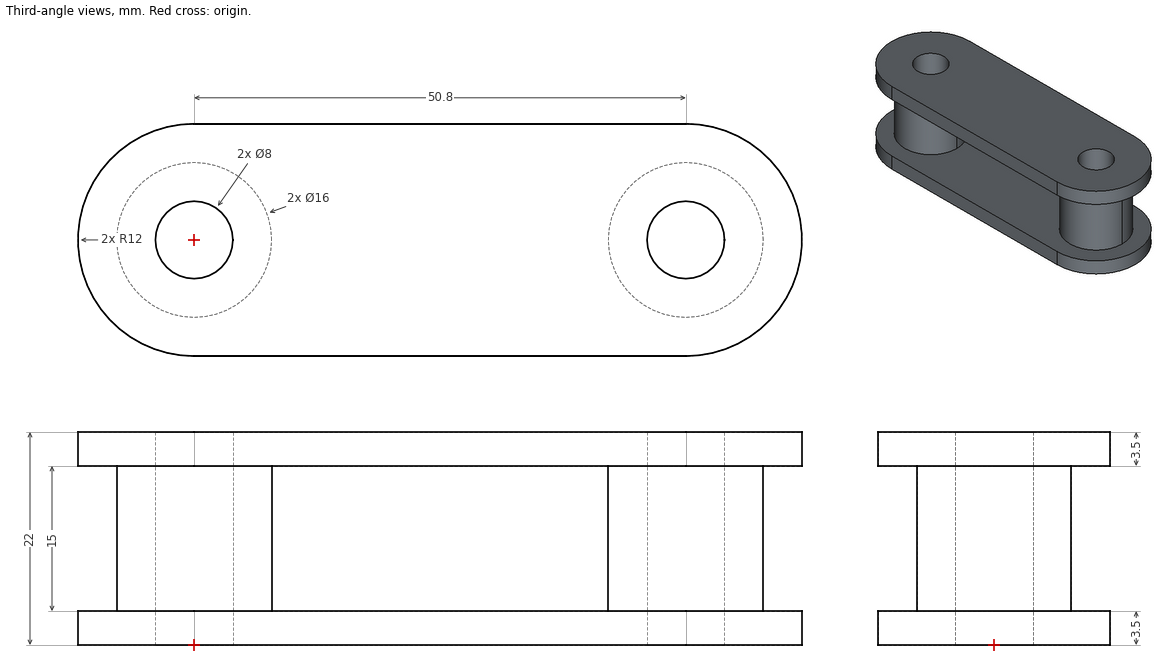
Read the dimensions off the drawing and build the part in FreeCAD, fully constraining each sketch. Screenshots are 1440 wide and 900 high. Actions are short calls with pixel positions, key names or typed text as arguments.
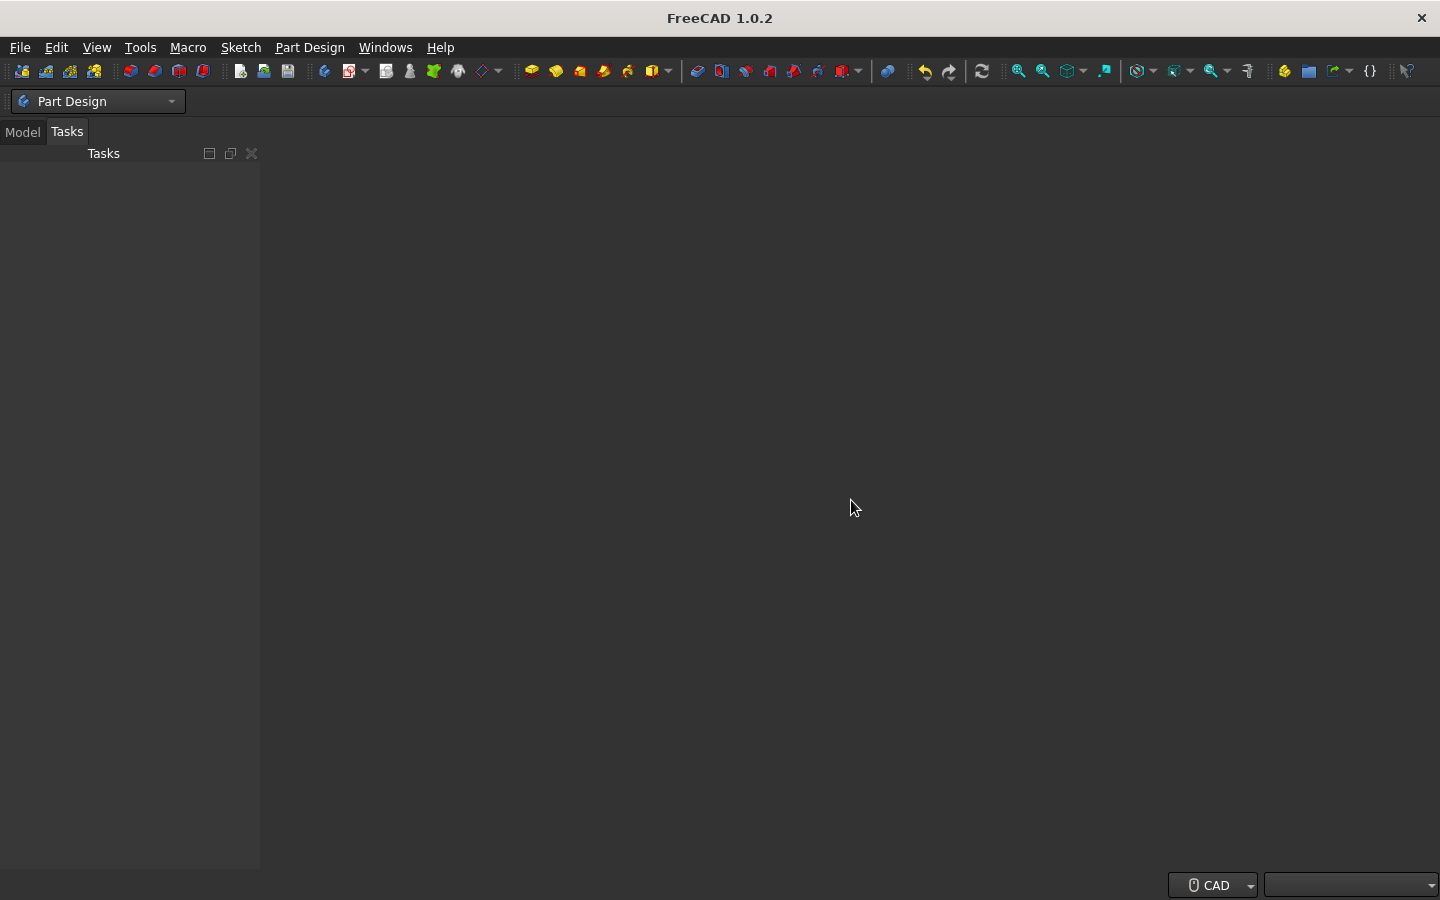
key(ctrl+n)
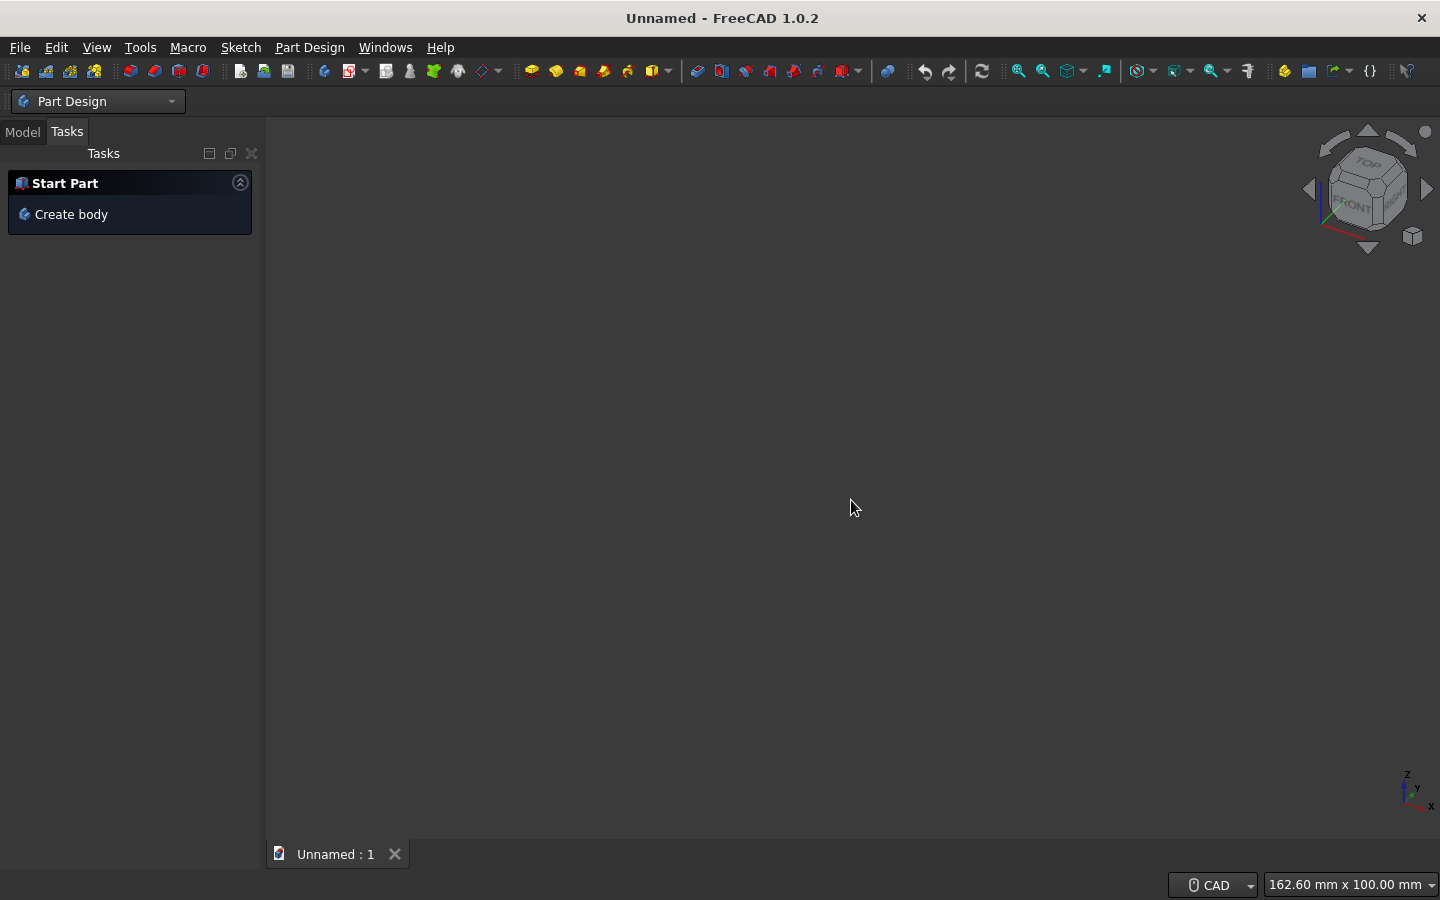
click(350, 72)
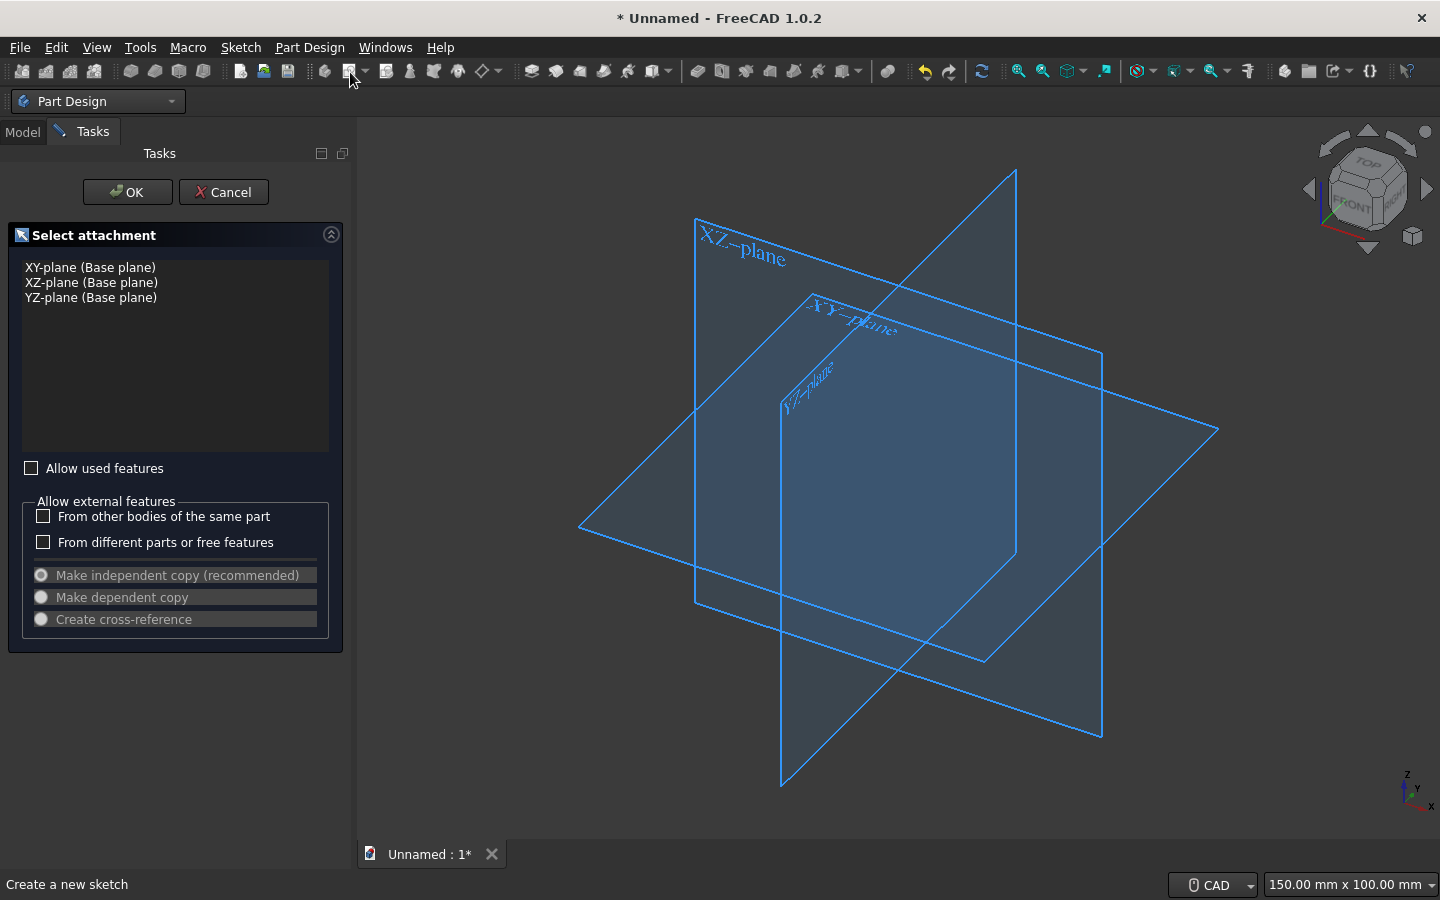
click(82, 268)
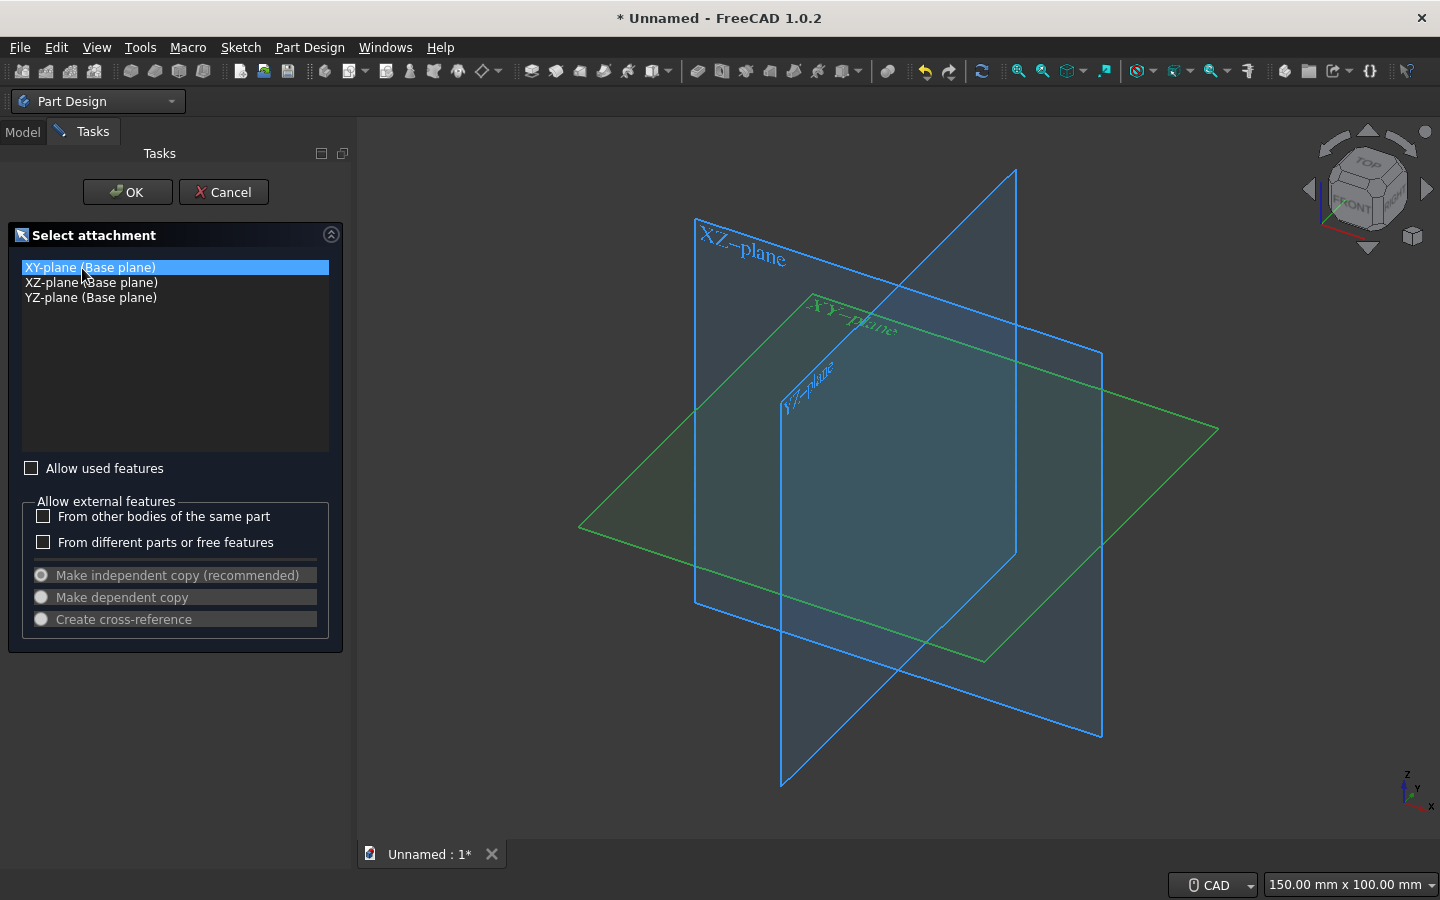
click(128, 192)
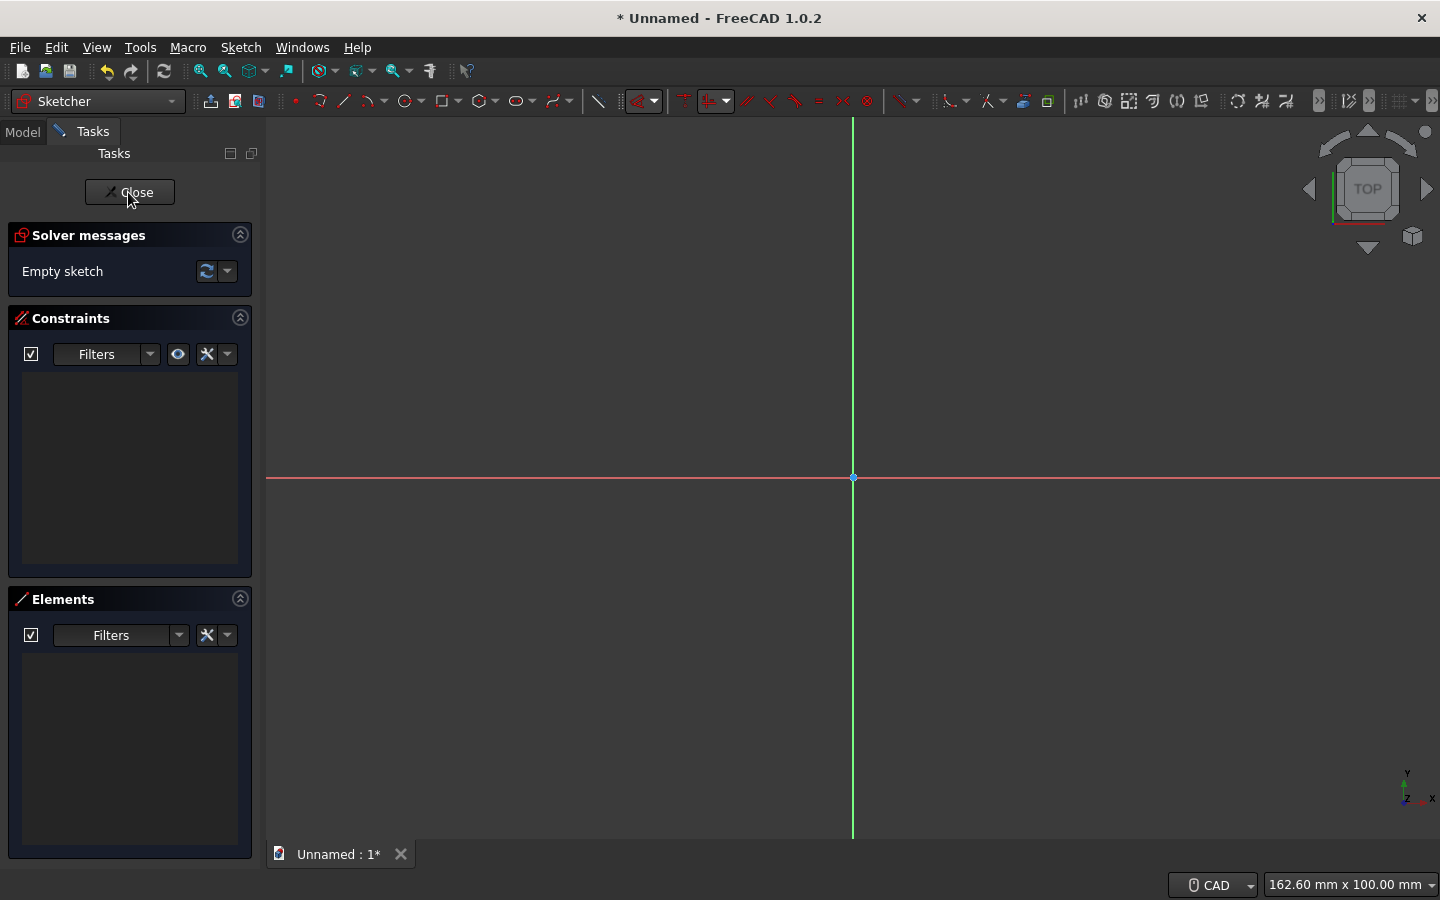
scroll(294, 478, down, 1)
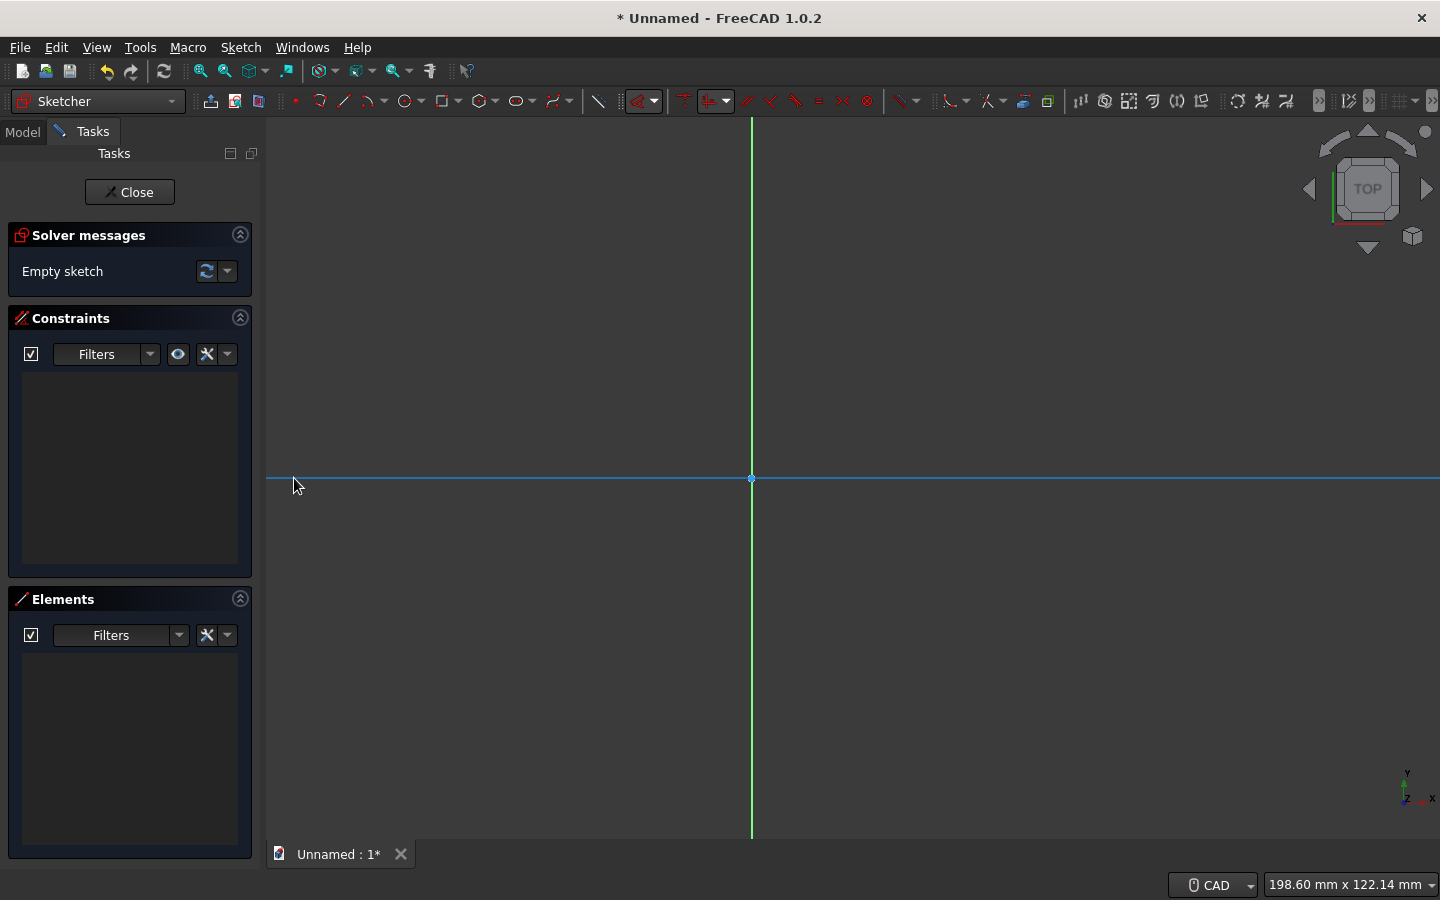
scroll(1140, 478, up, 2)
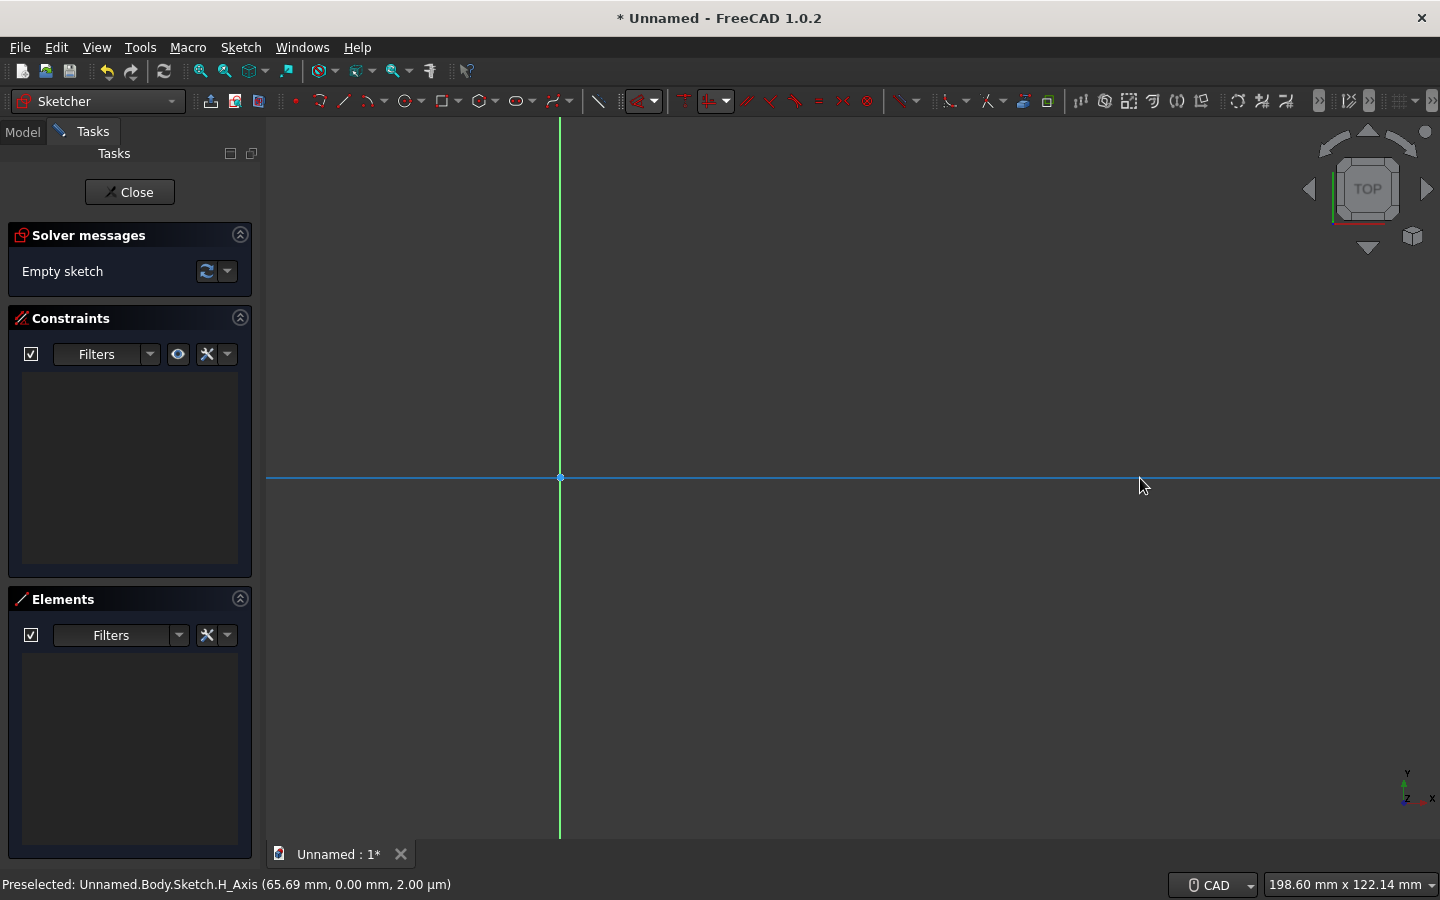
click(516, 102)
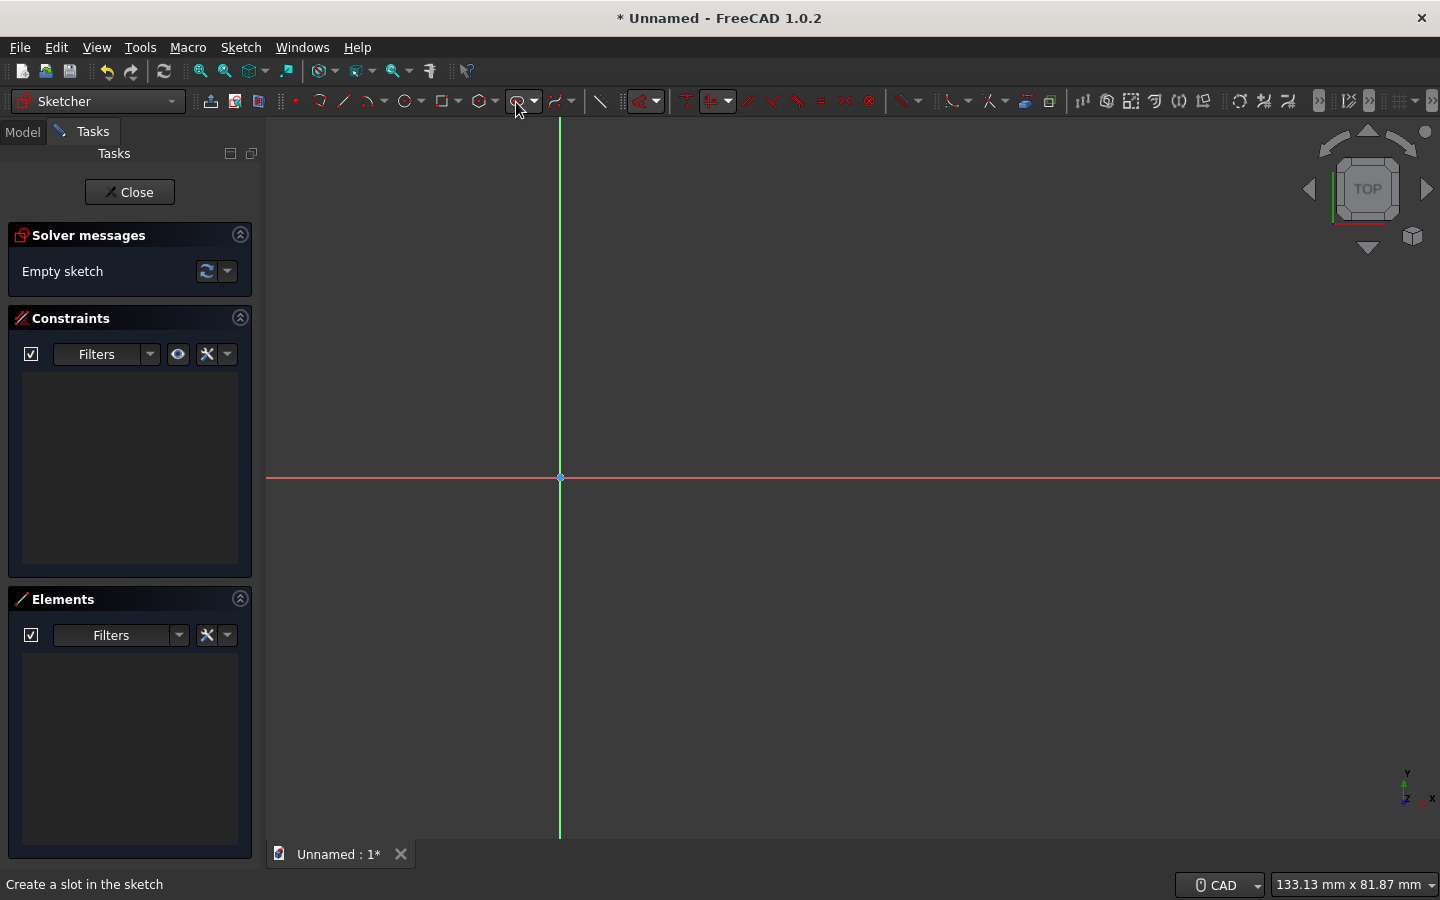
click(560, 478)